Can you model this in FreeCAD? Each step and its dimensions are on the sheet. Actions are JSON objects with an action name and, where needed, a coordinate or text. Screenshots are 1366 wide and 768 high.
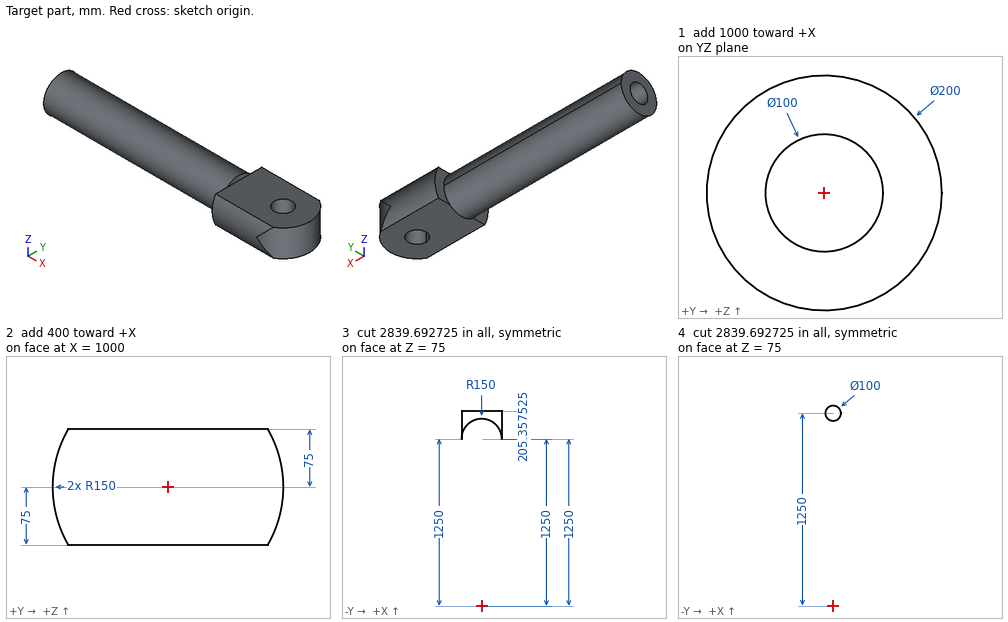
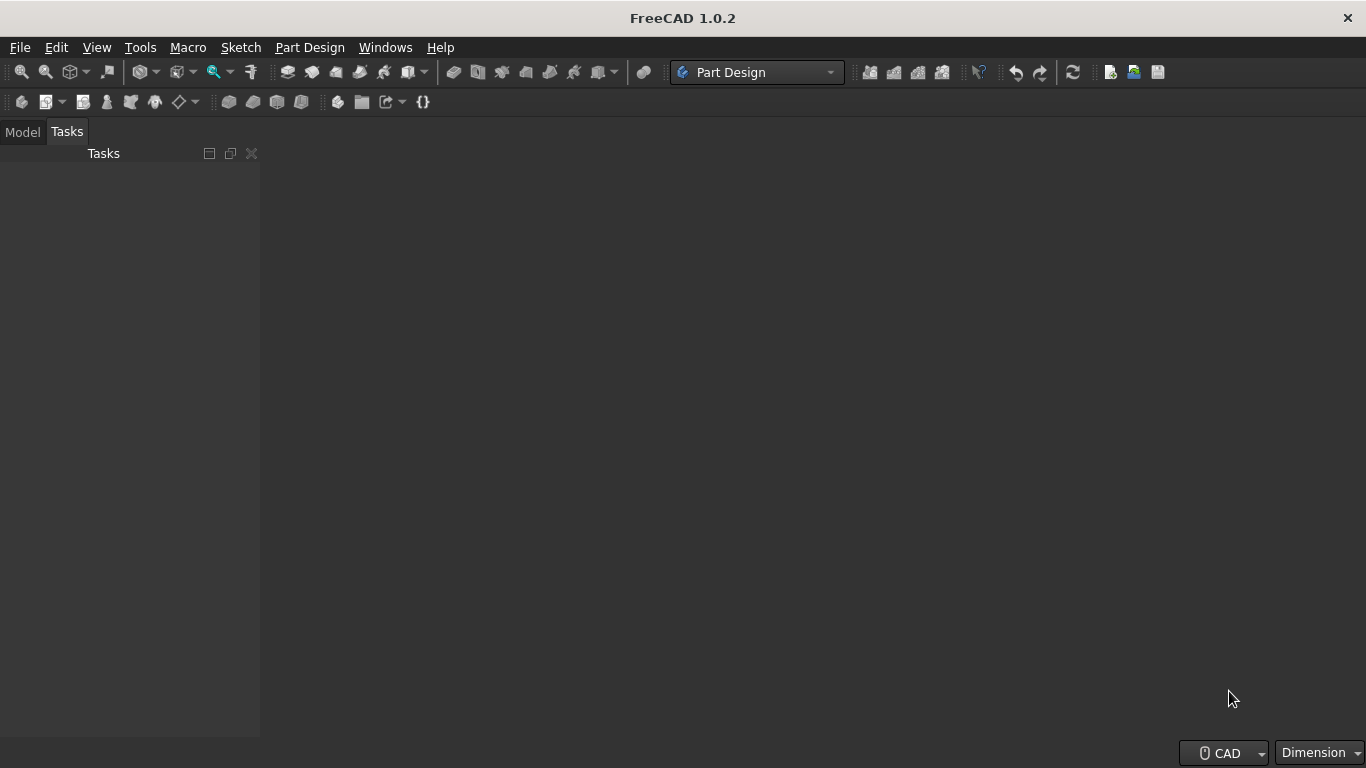
{"action": "left_click", "coordinate": [1110, 72]}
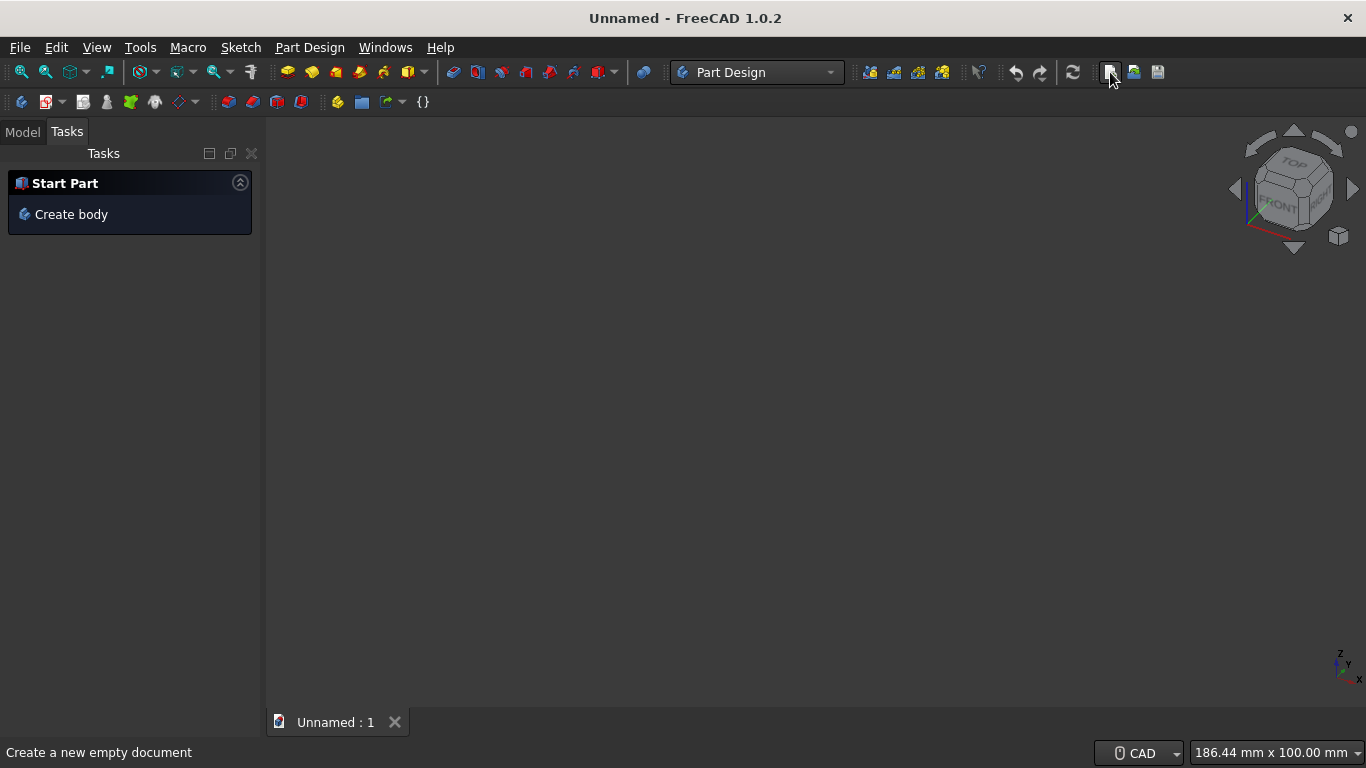
{"action": "left_click", "coordinate": [46, 102]}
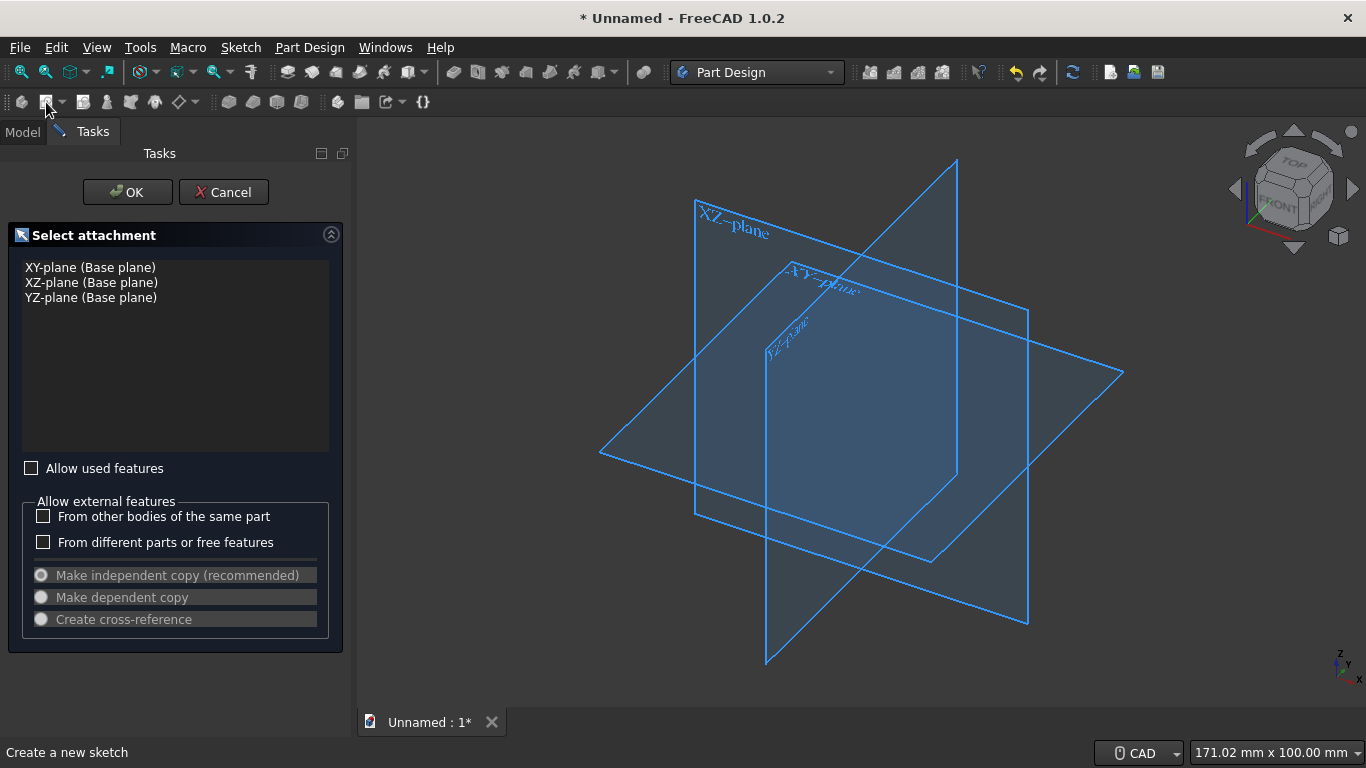
{"action": "left_click", "coordinate": [82, 298]}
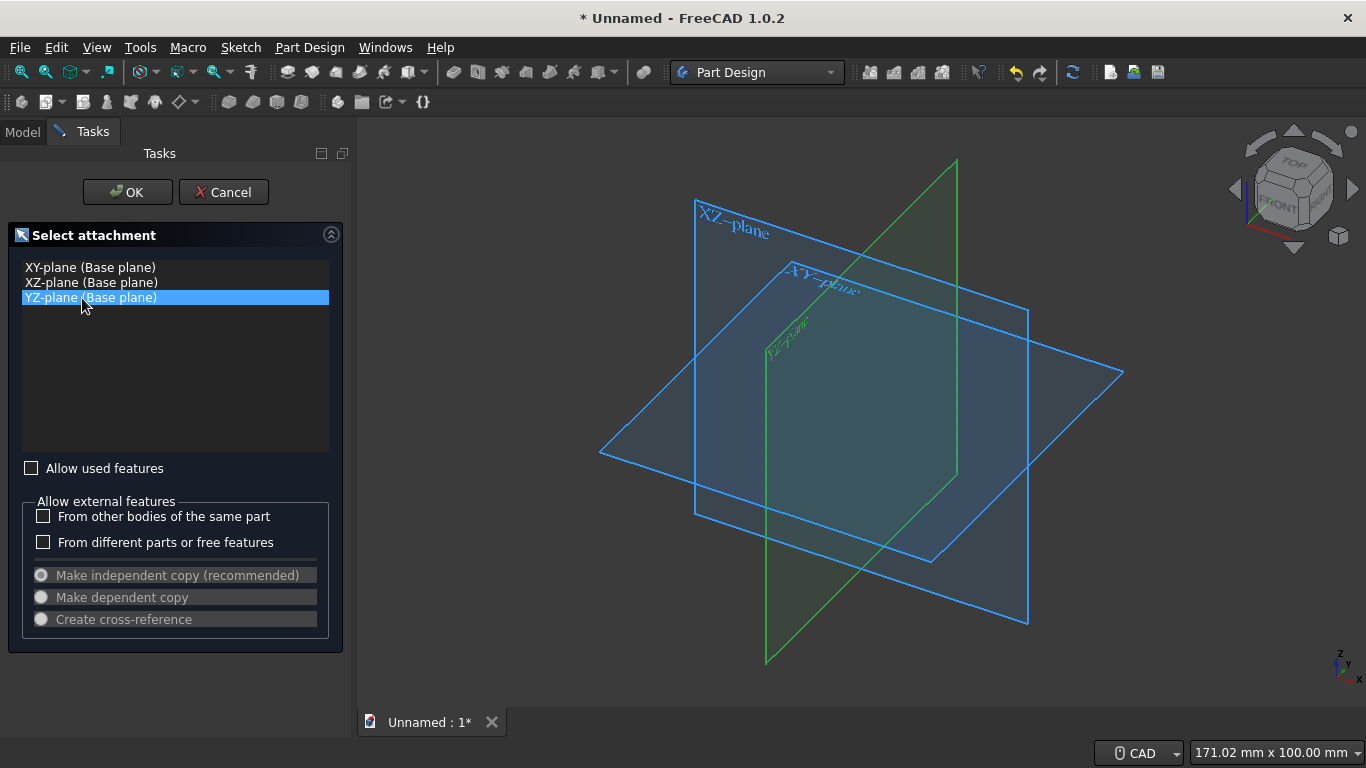
{"action": "left_click", "coordinate": [128, 192]}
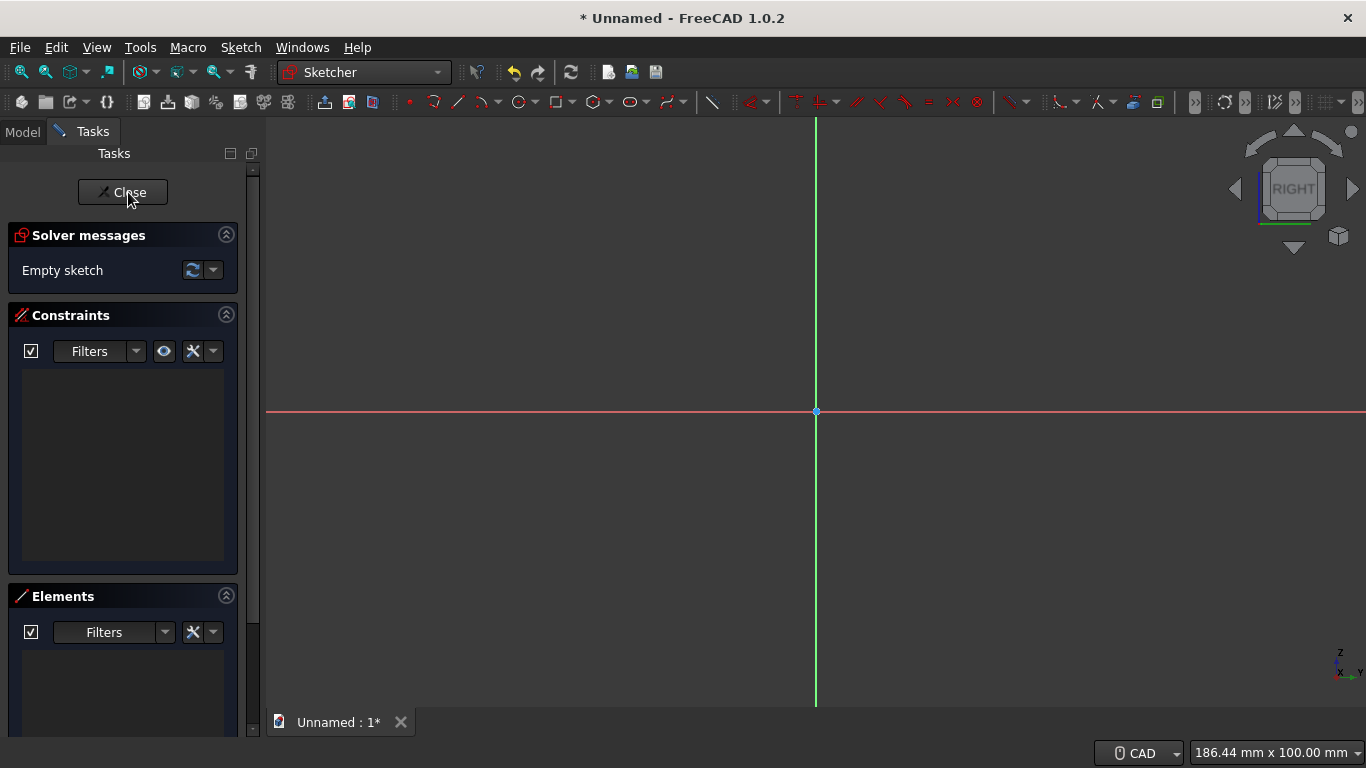
{"action": "scroll", "coordinate": [718, 412], "scroll_direction": "down", "scroll_amount": 6}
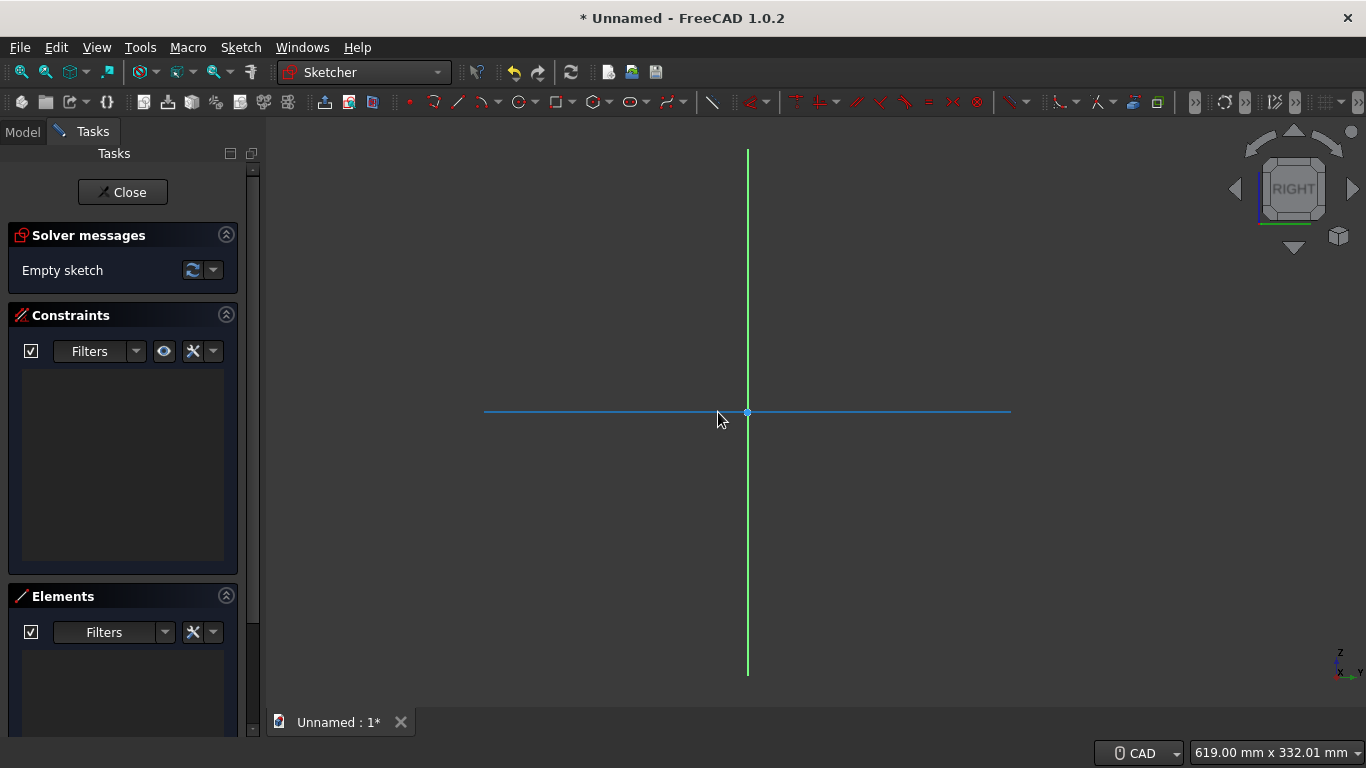
{"action": "left_click", "coordinate": [520, 102]}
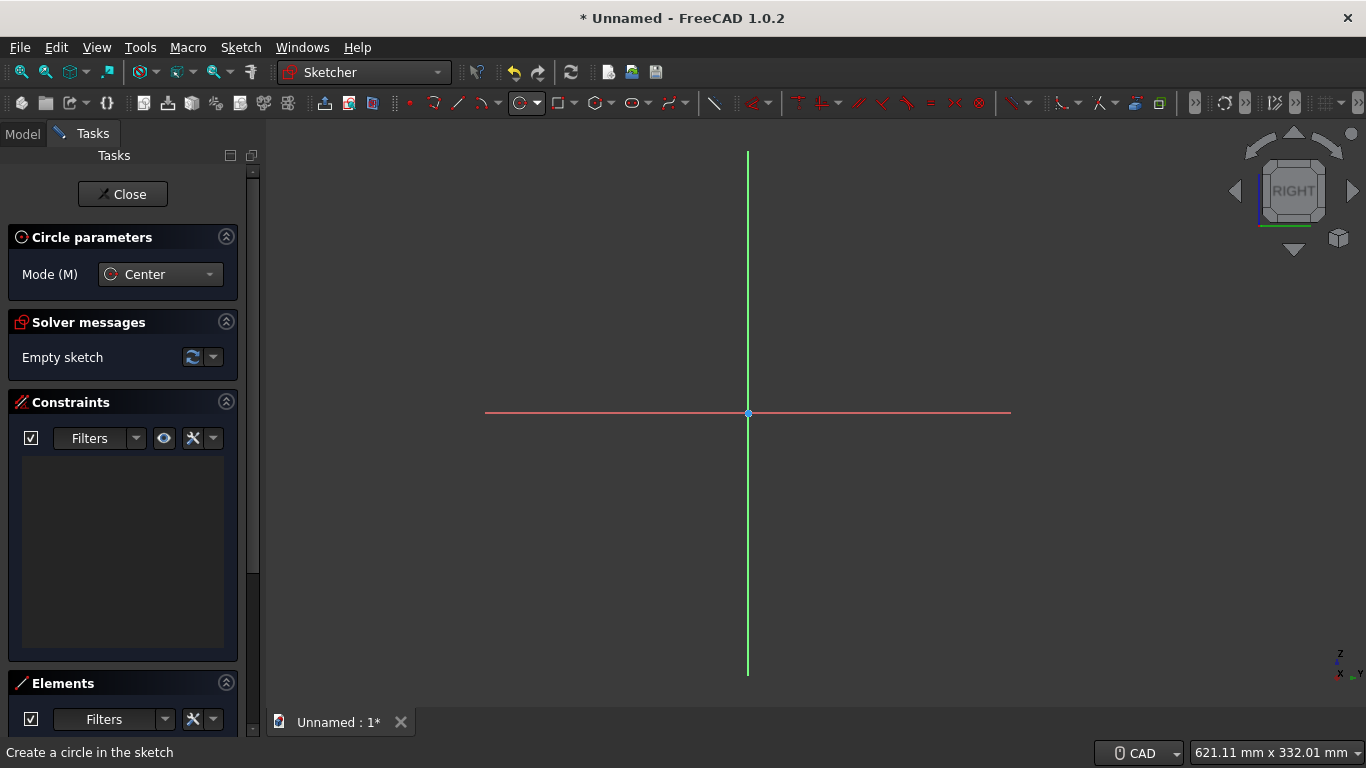
{"action": "left_click", "coordinate": [748, 413]}
{"action": "mouse_move", "coordinate": [873, 288]}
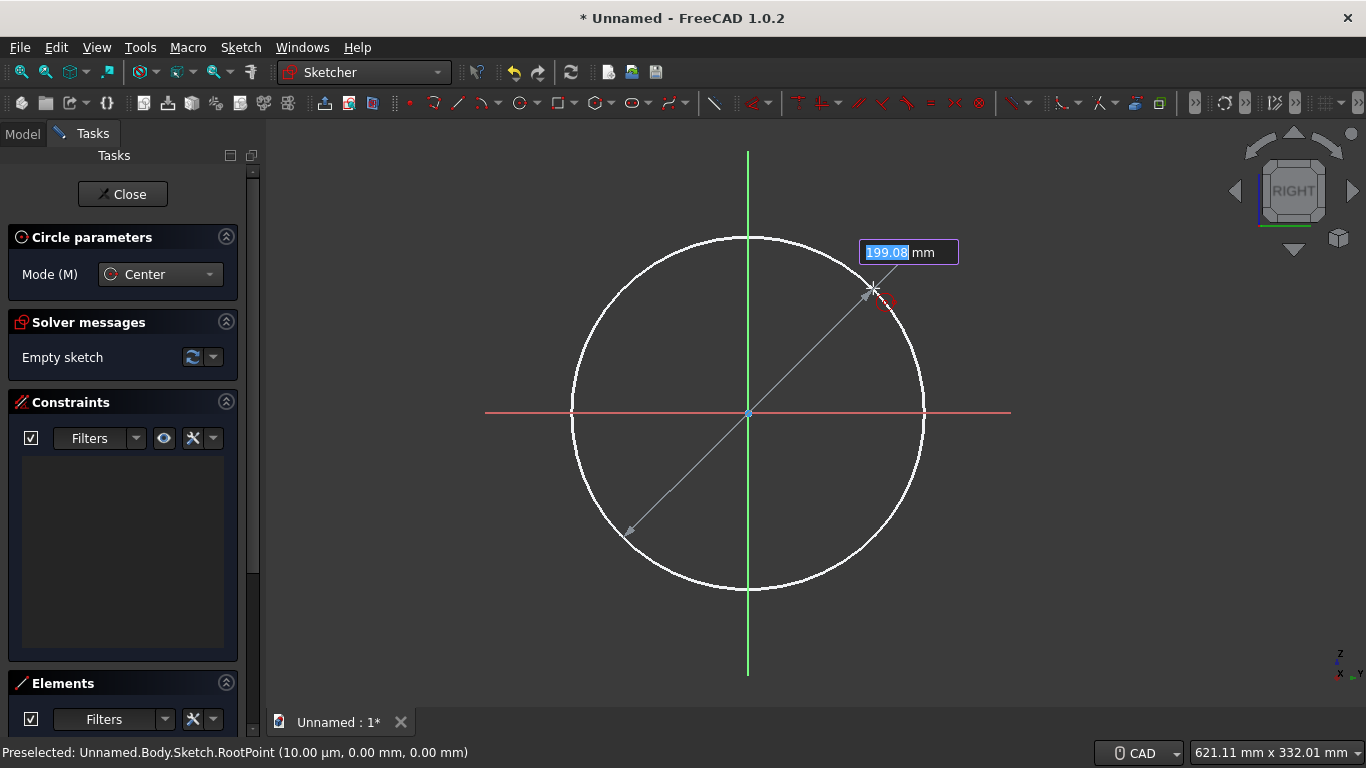
{"action": "type", "text": "200"}
{"action": "key", "text": "Return"}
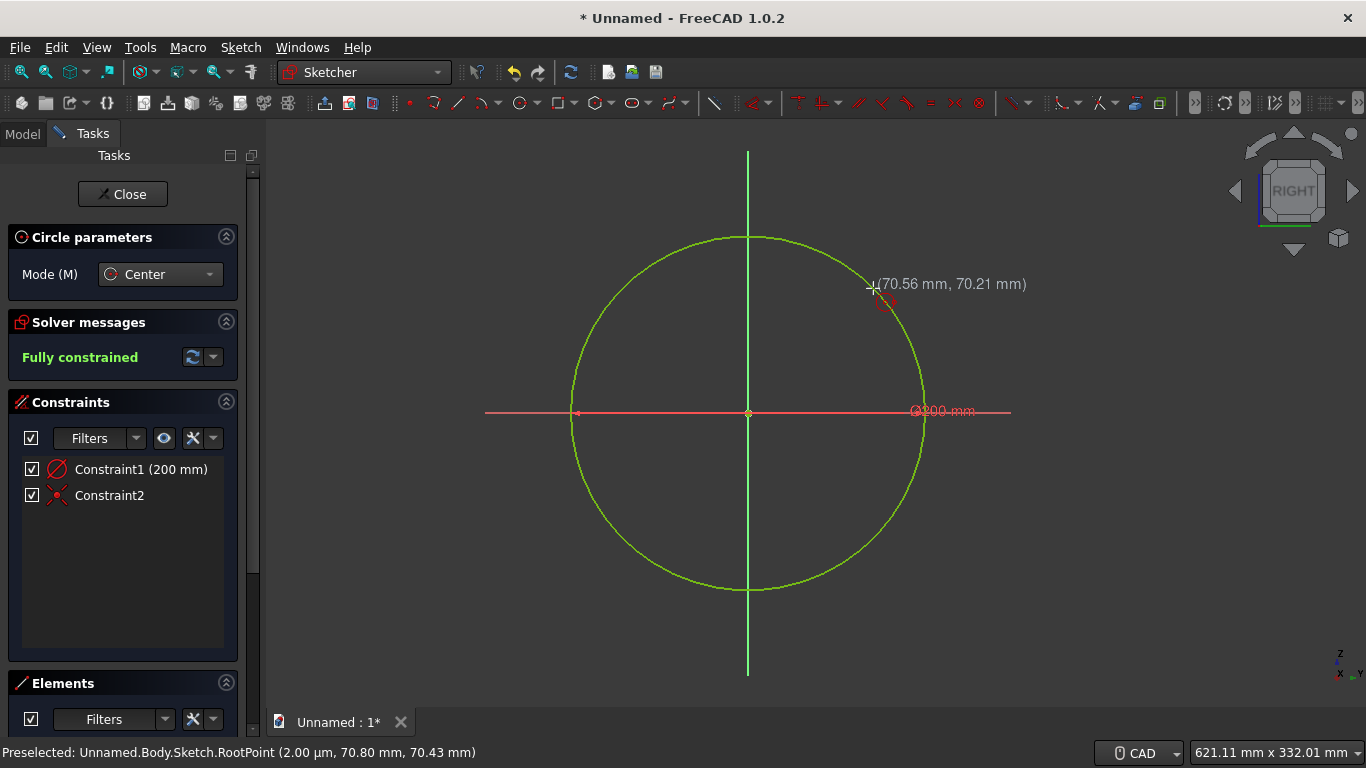
{"action": "left_click", "coordinate": [748, 413]}
{"action": "mouse_move", "coordinate": [811, 351]}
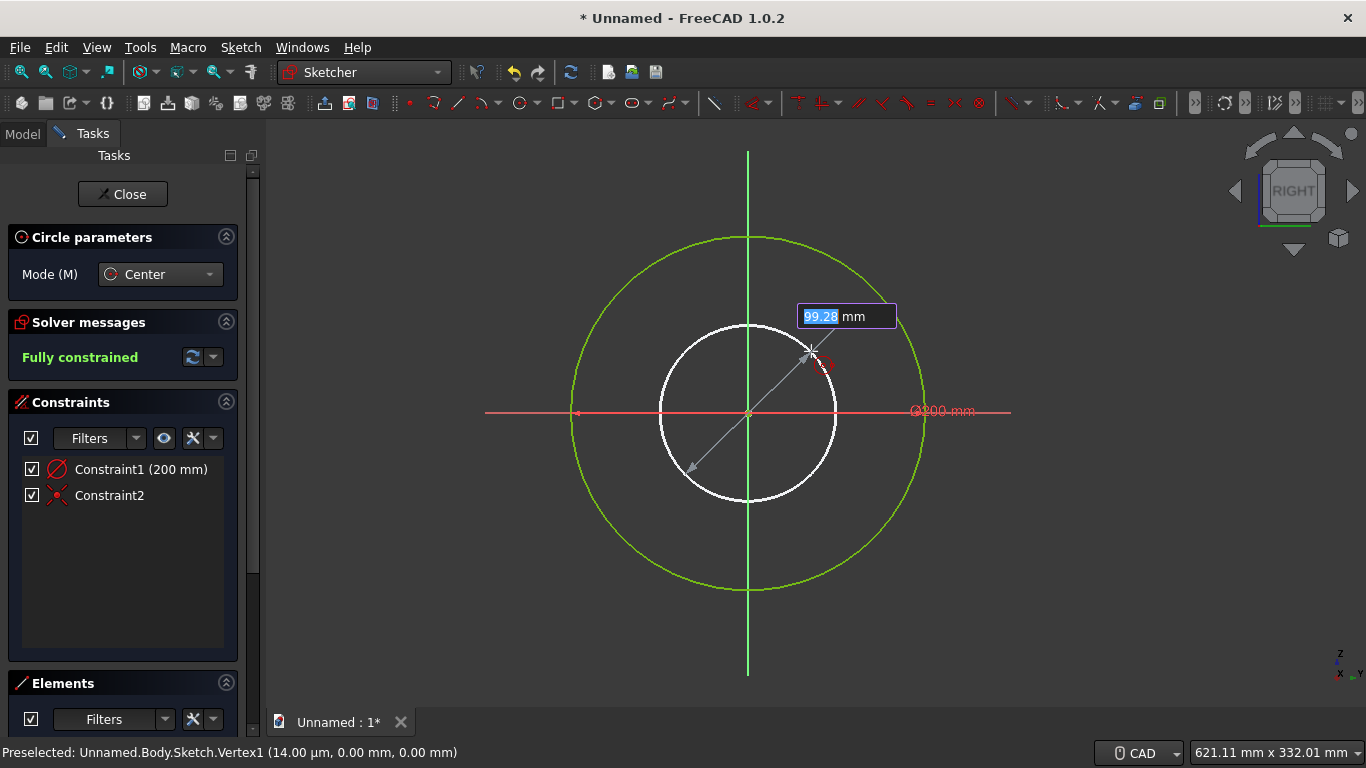
{"action": "type", "text": "100"}
{"action": "key", "text": "Return"}
{"action": "key", "text": "Escape"}